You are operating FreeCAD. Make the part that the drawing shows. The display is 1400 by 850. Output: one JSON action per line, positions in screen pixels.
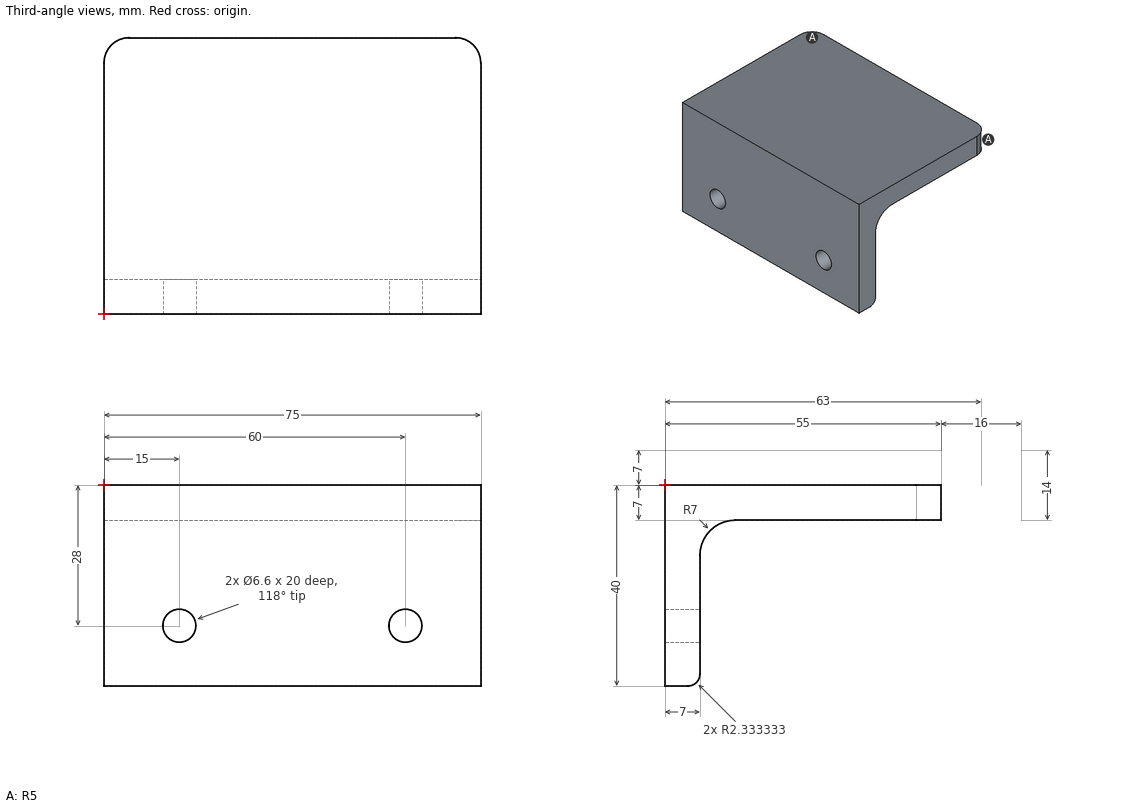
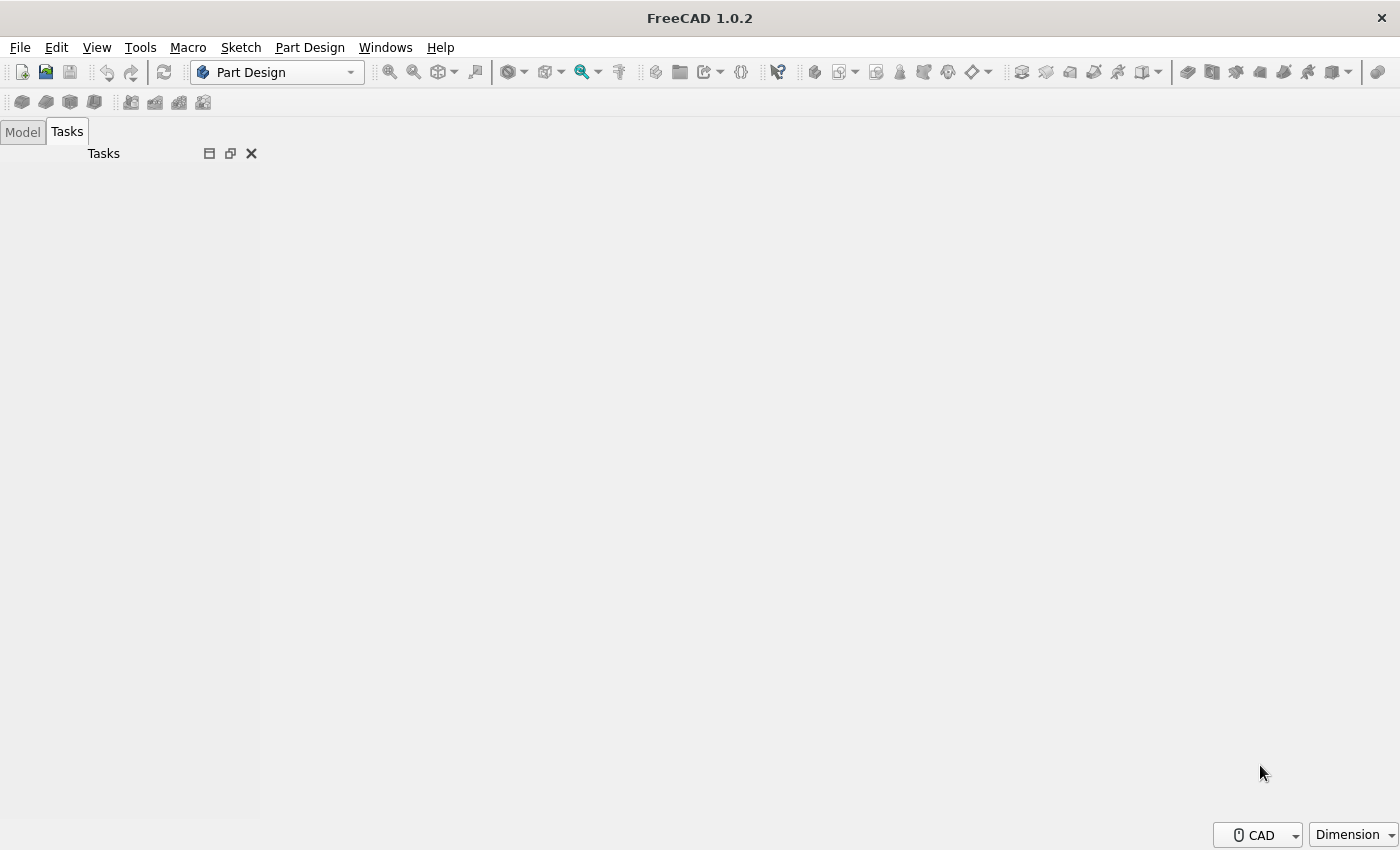
{"action": "key", "text": "ctrl+n"}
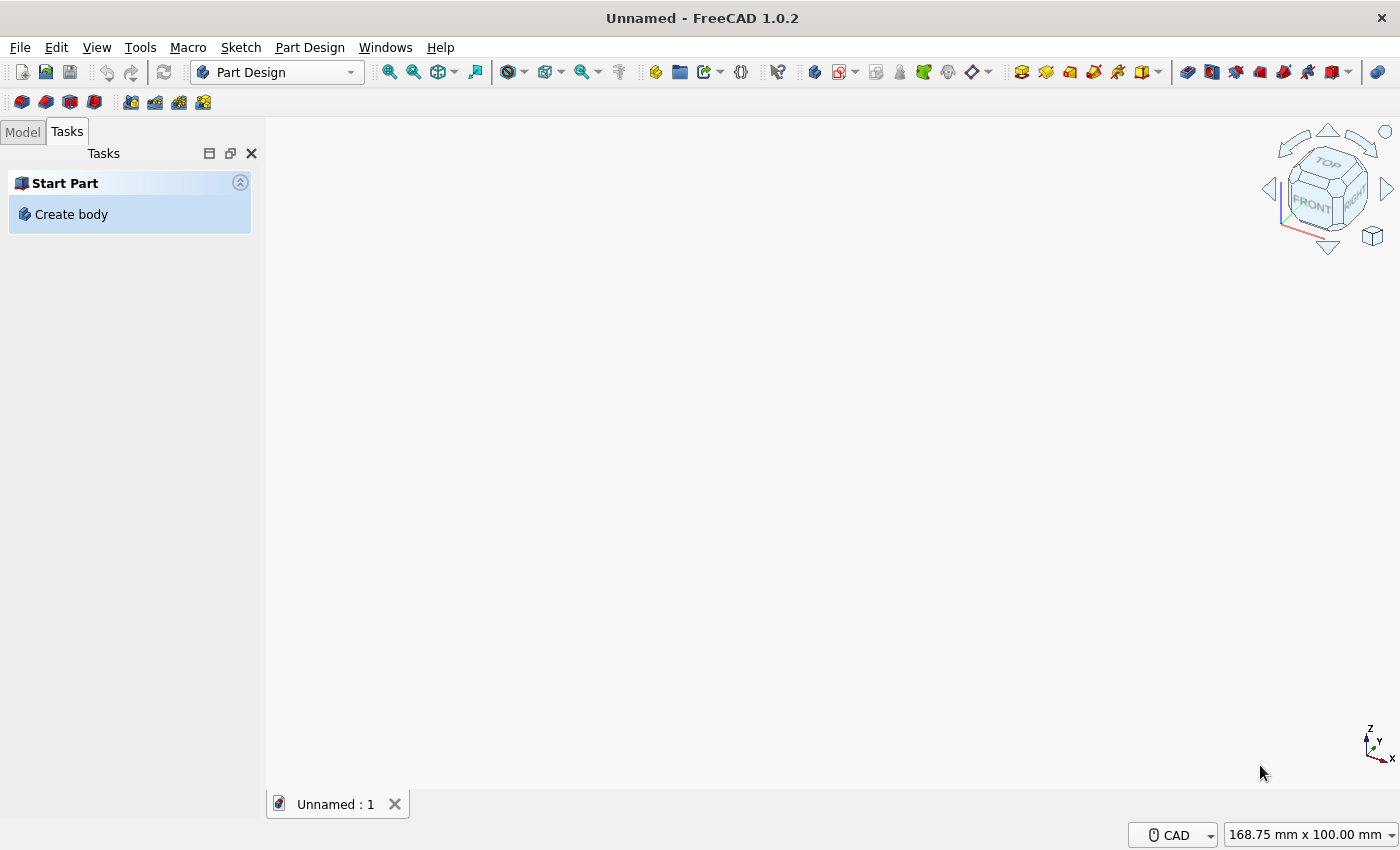
{"action": "left_click", "coordinate": [840, 72]}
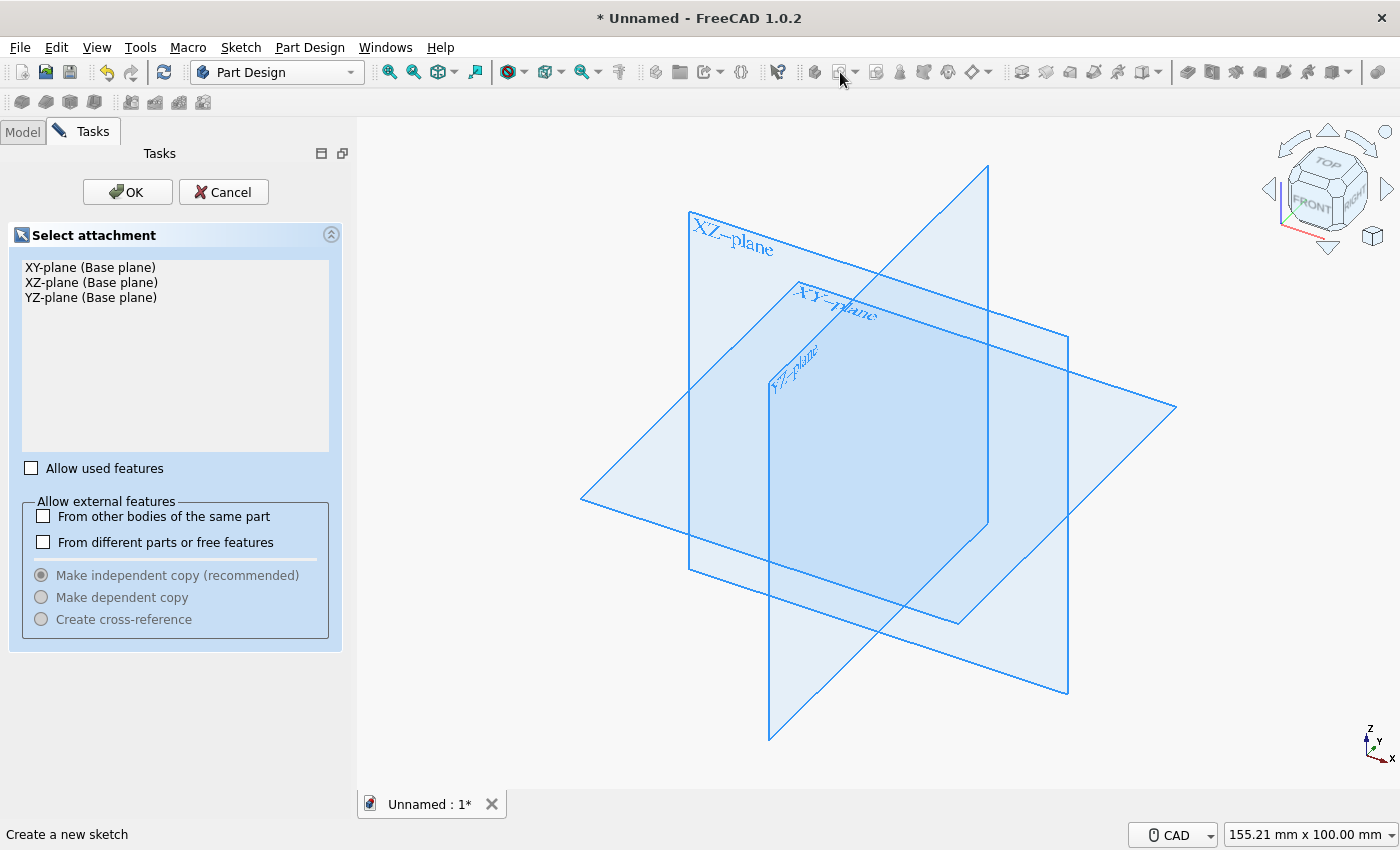
{"action": "left_click", "coordinate": [82, 298]}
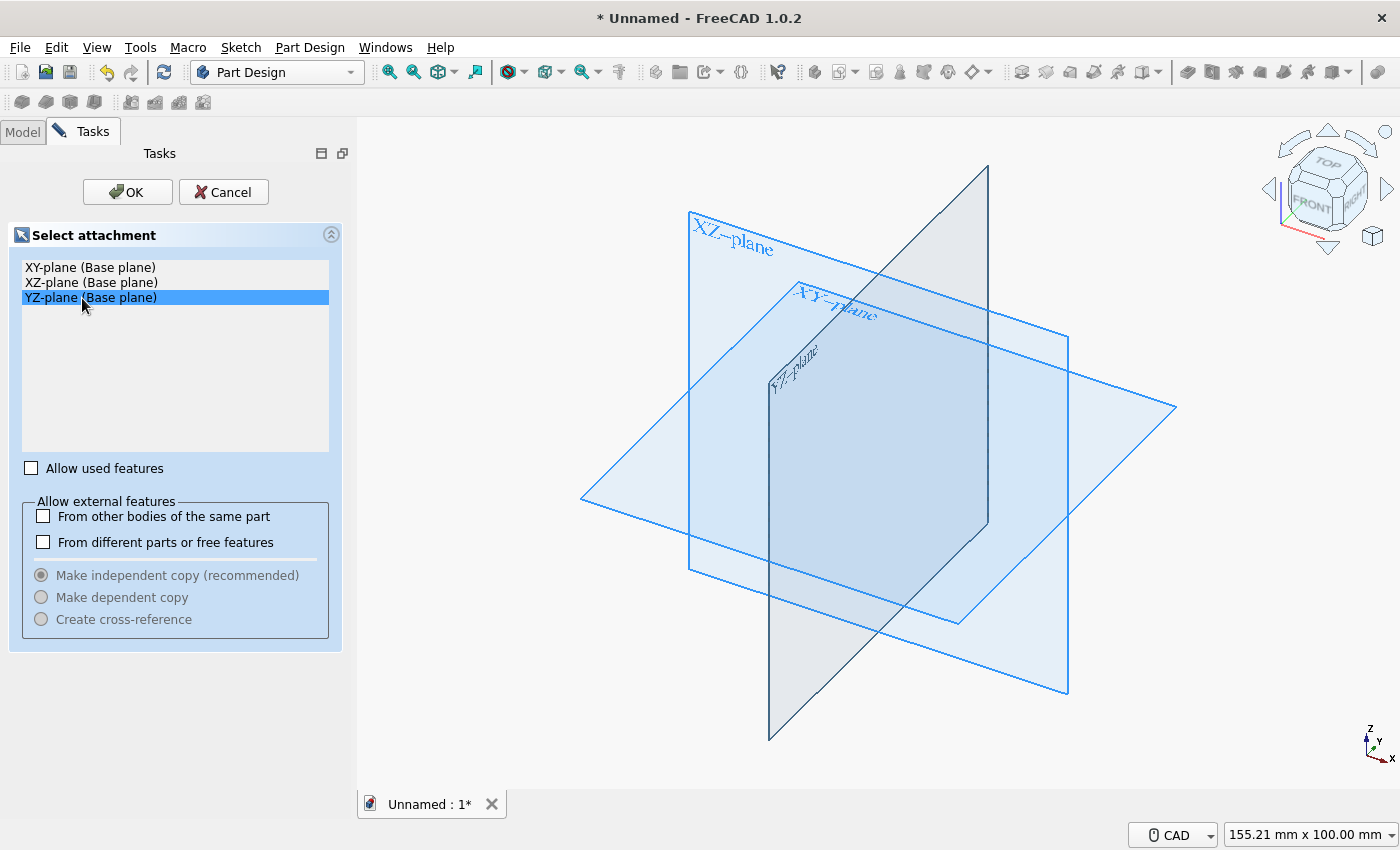
{"action": "left_click", "coordinate": [128, 192]}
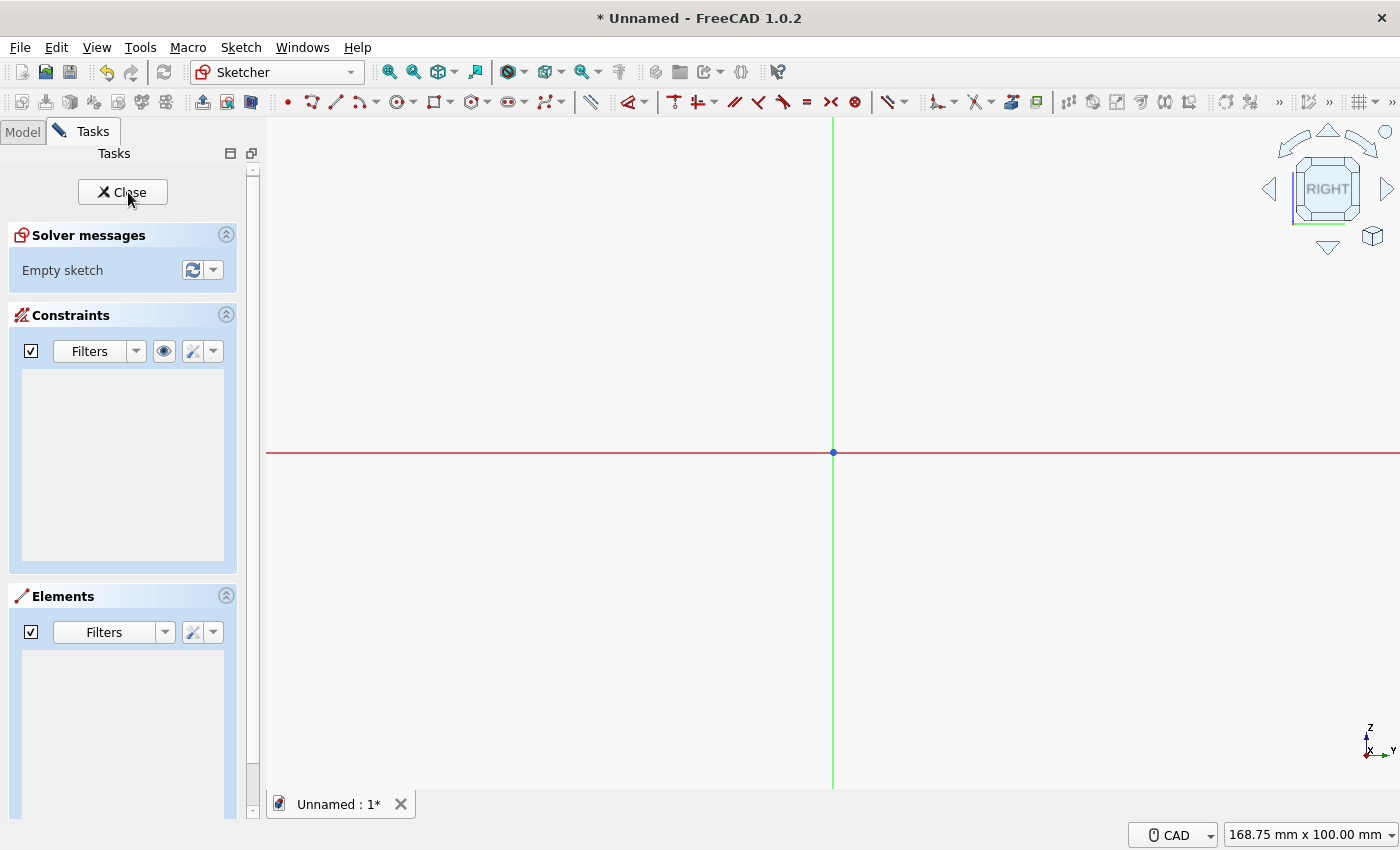
{"action": "scroll", "coordinate": [294, 145], "scroll_direction": "down", "scroll_amount": 1}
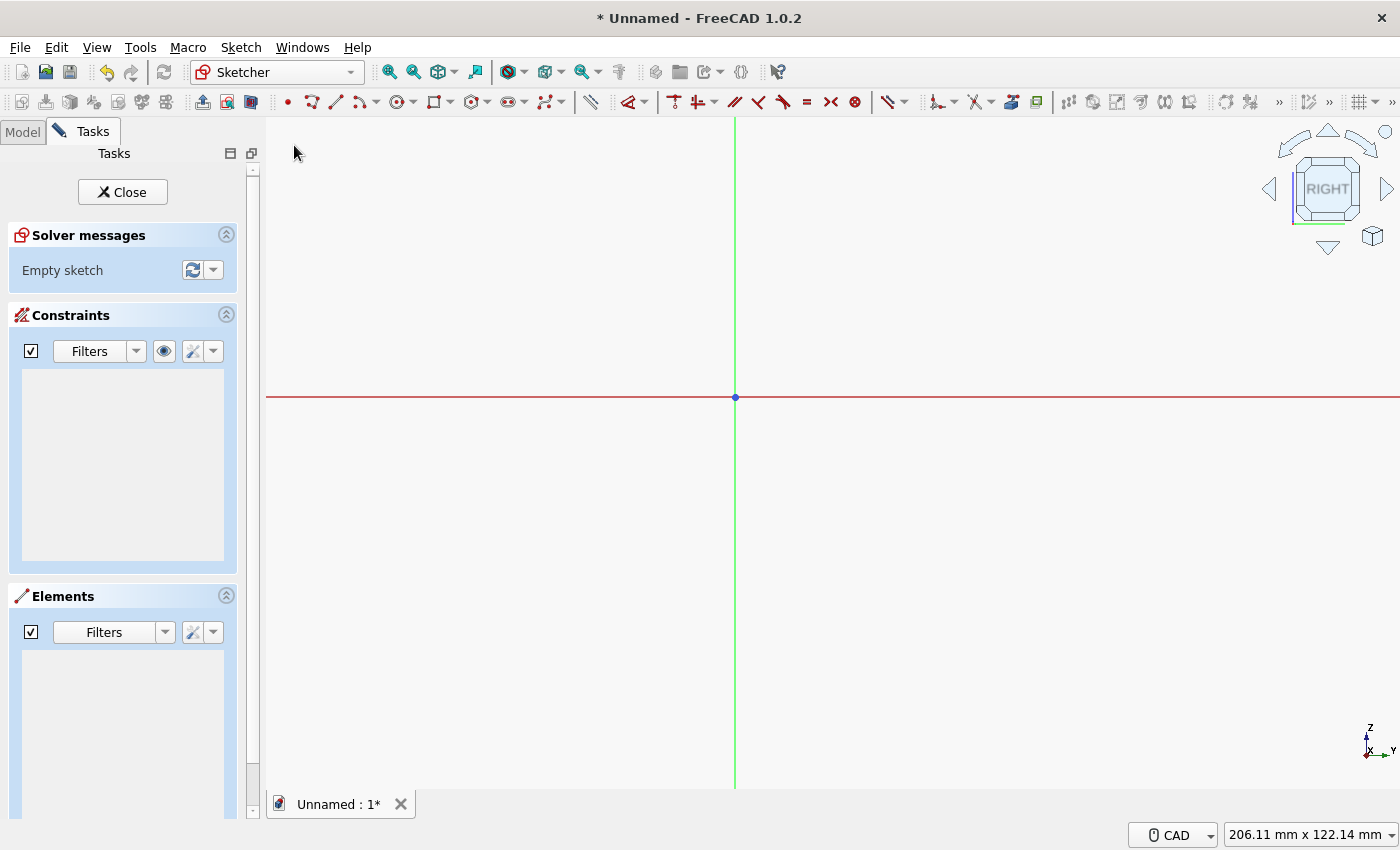
{"action": "scroll", "coordinate": [1084, 573], "scroll_direction": "up", "scroll_amount": 3}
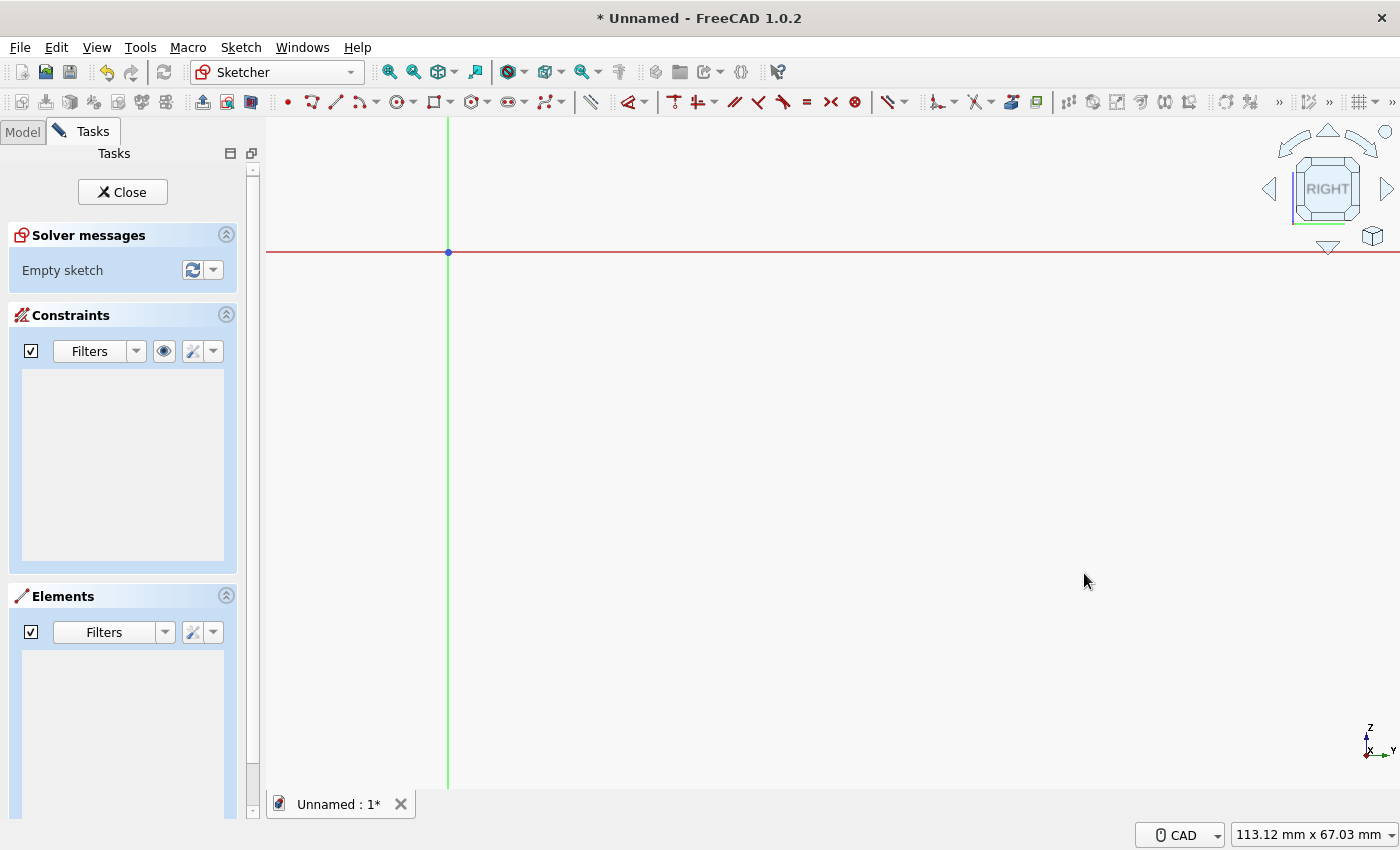
{"action": "left_click", "coordinate": [336, 102]}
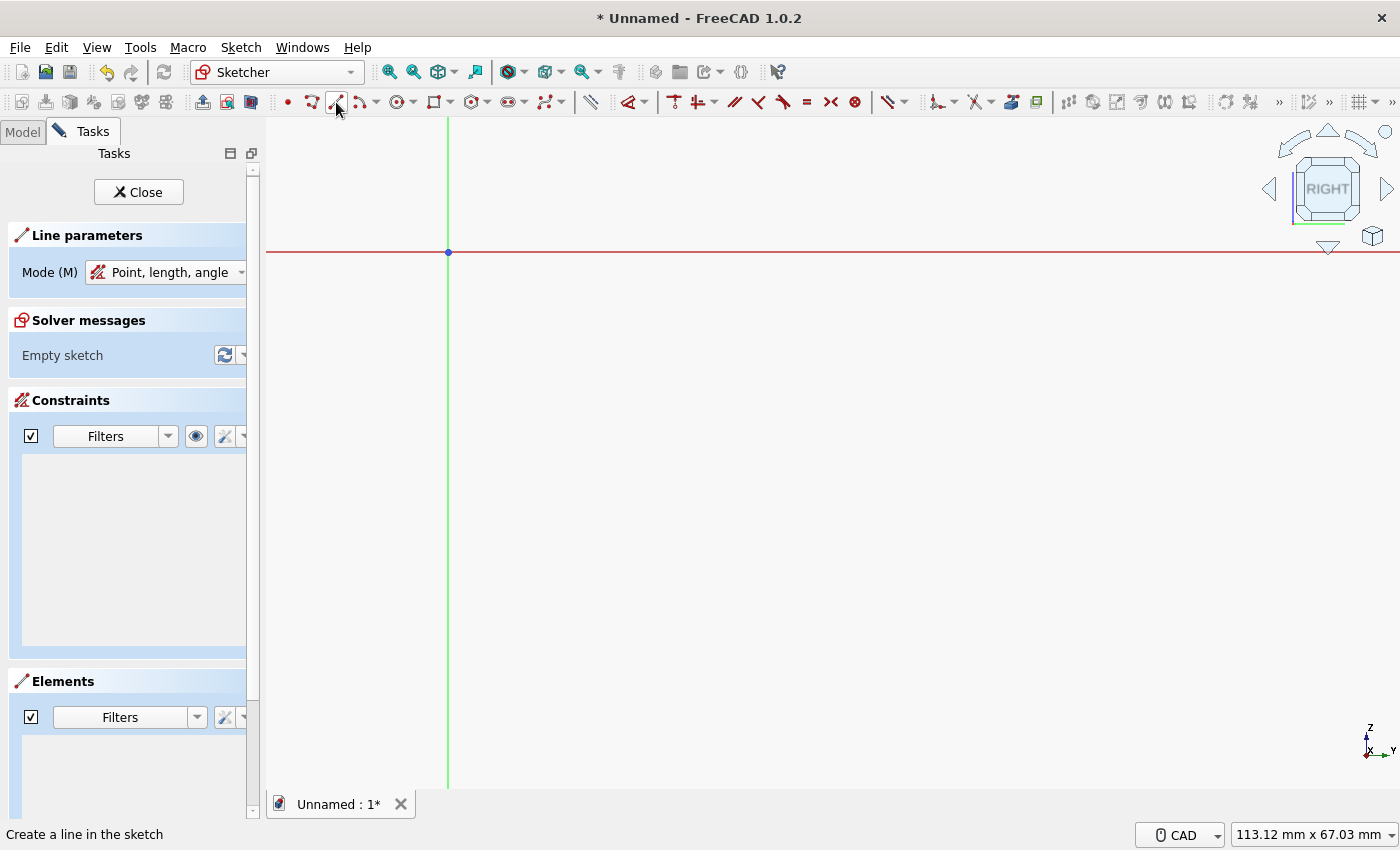
{"action": "left_click", "coordinate": [518, 630]}
{"action": "left_click", "coordinate": [518, 392]}